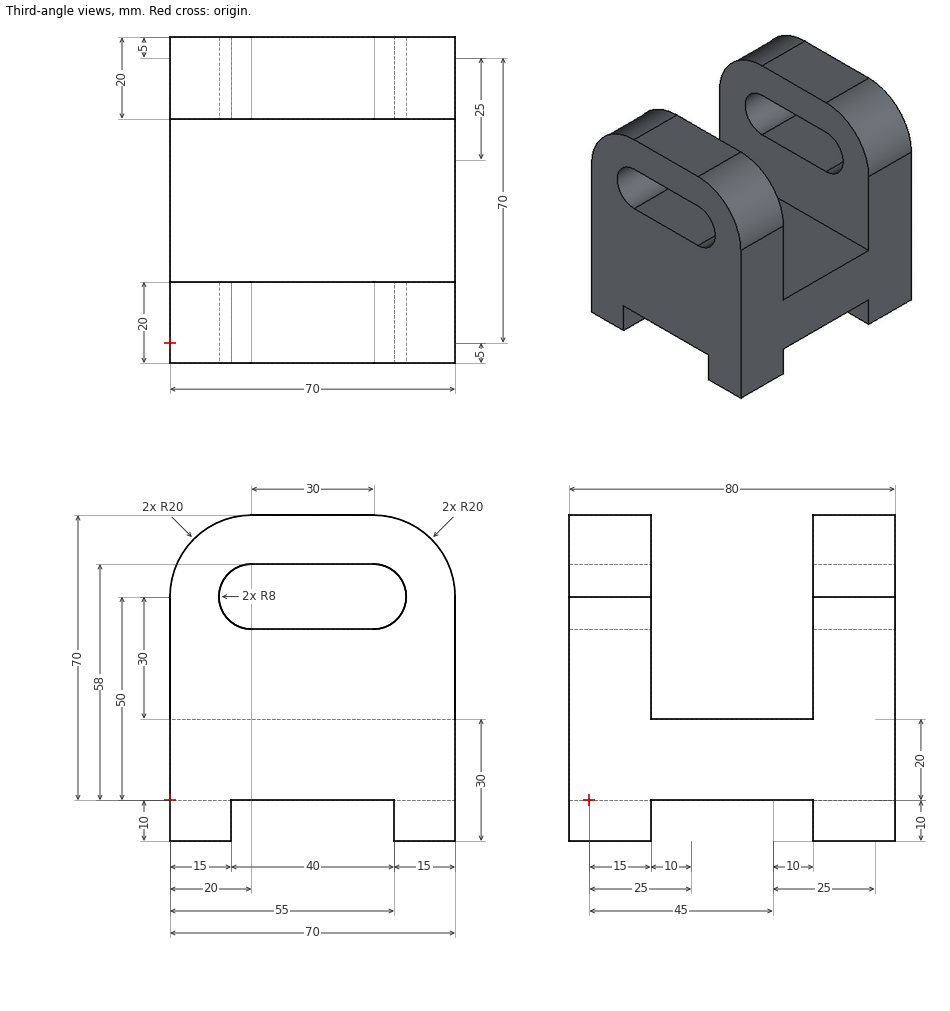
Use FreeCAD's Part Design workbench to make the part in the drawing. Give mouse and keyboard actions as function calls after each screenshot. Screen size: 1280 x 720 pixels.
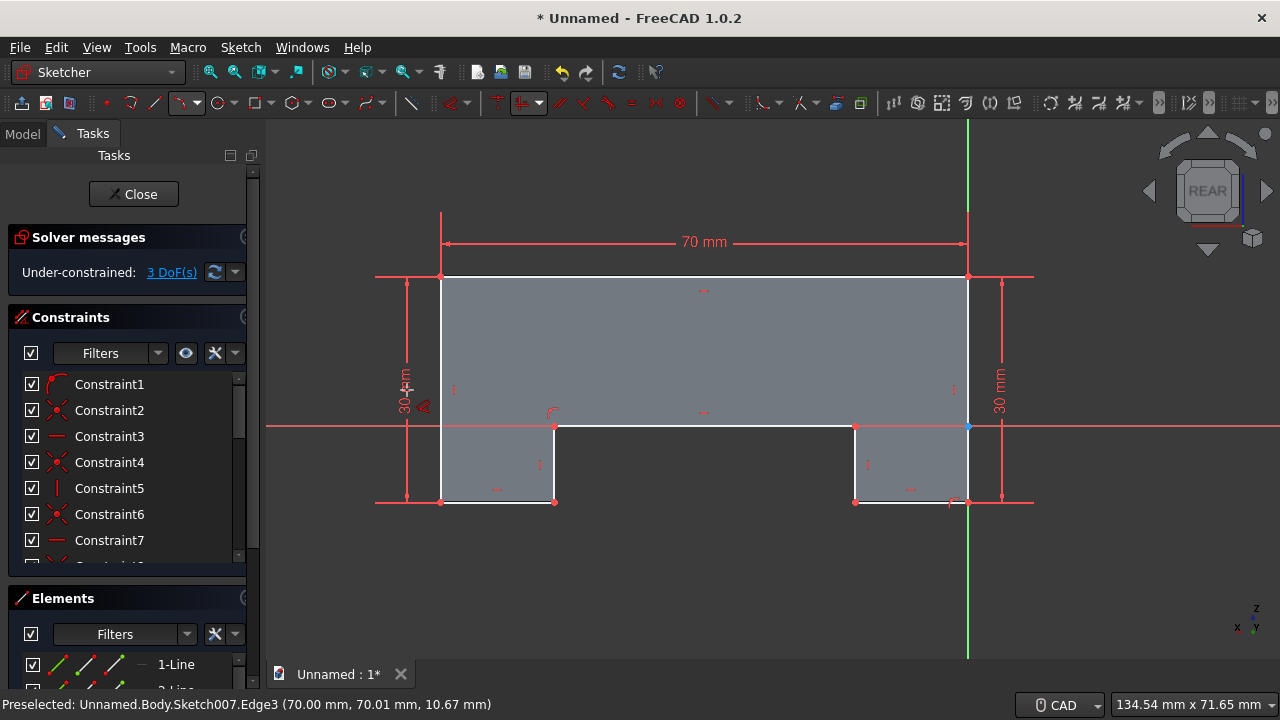
click(475, 503)
click(497, 537)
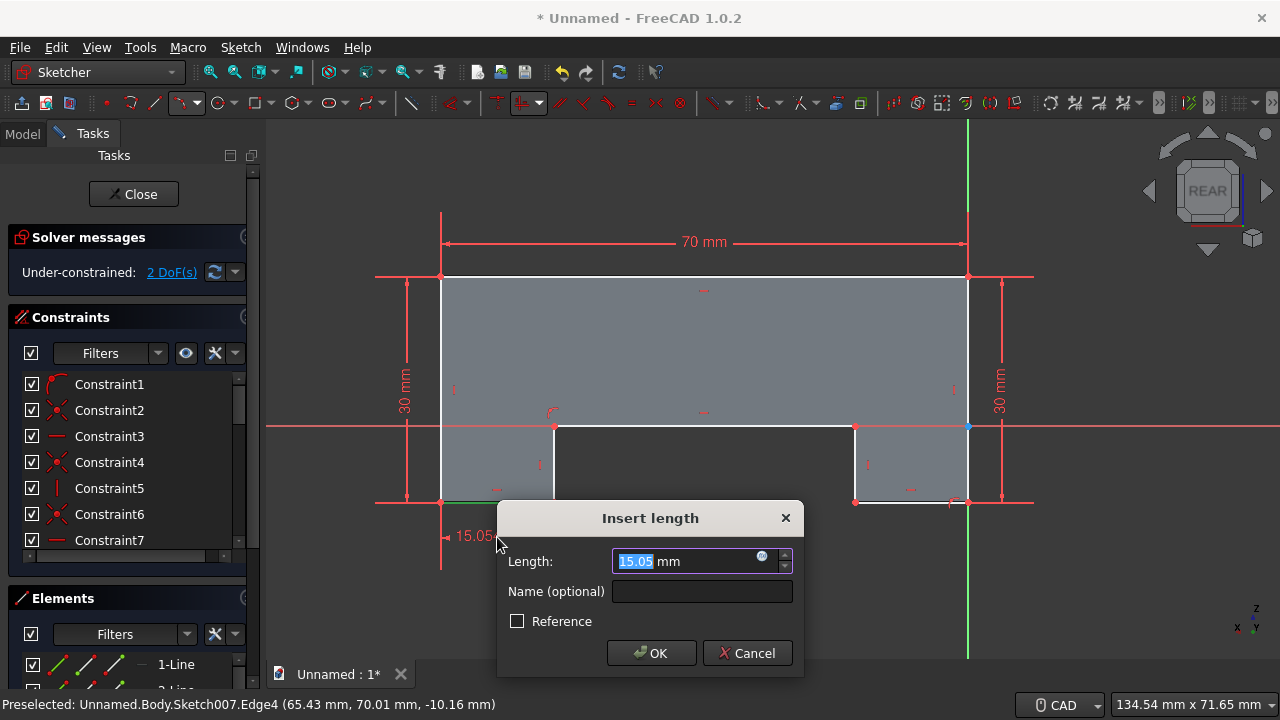
text(15)
key(Return)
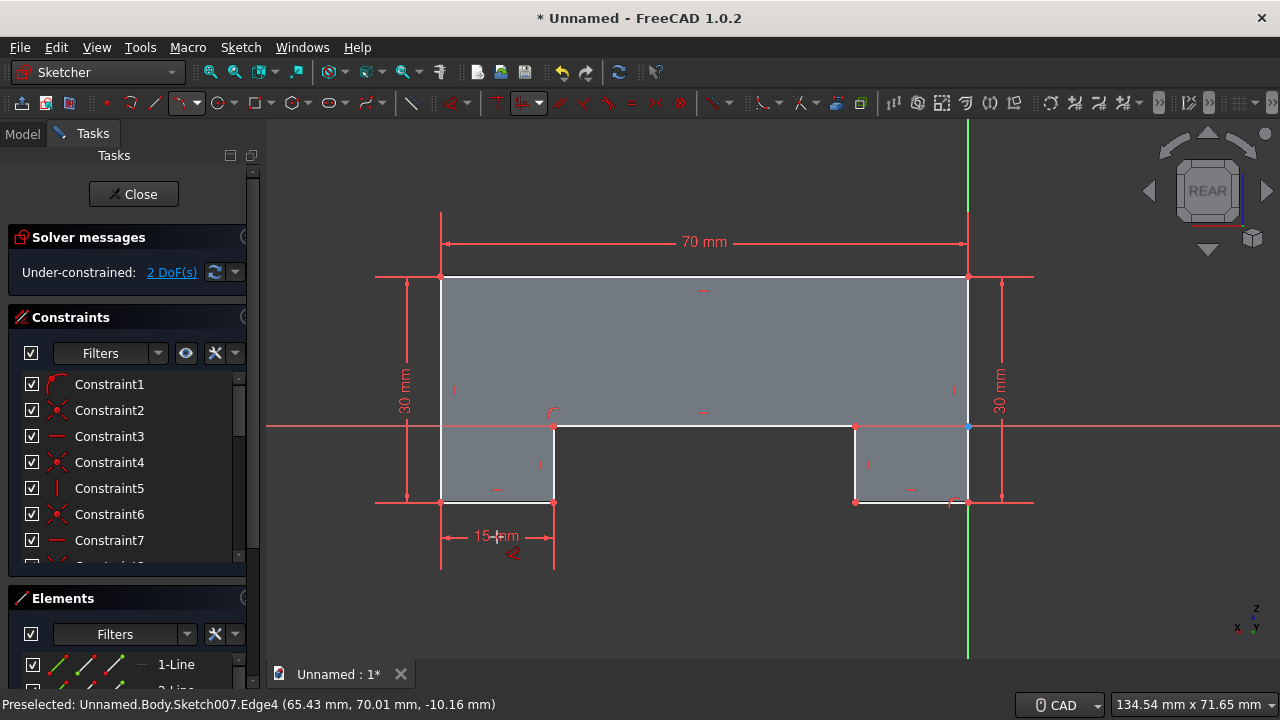
click(554, 480)
click(520, 465)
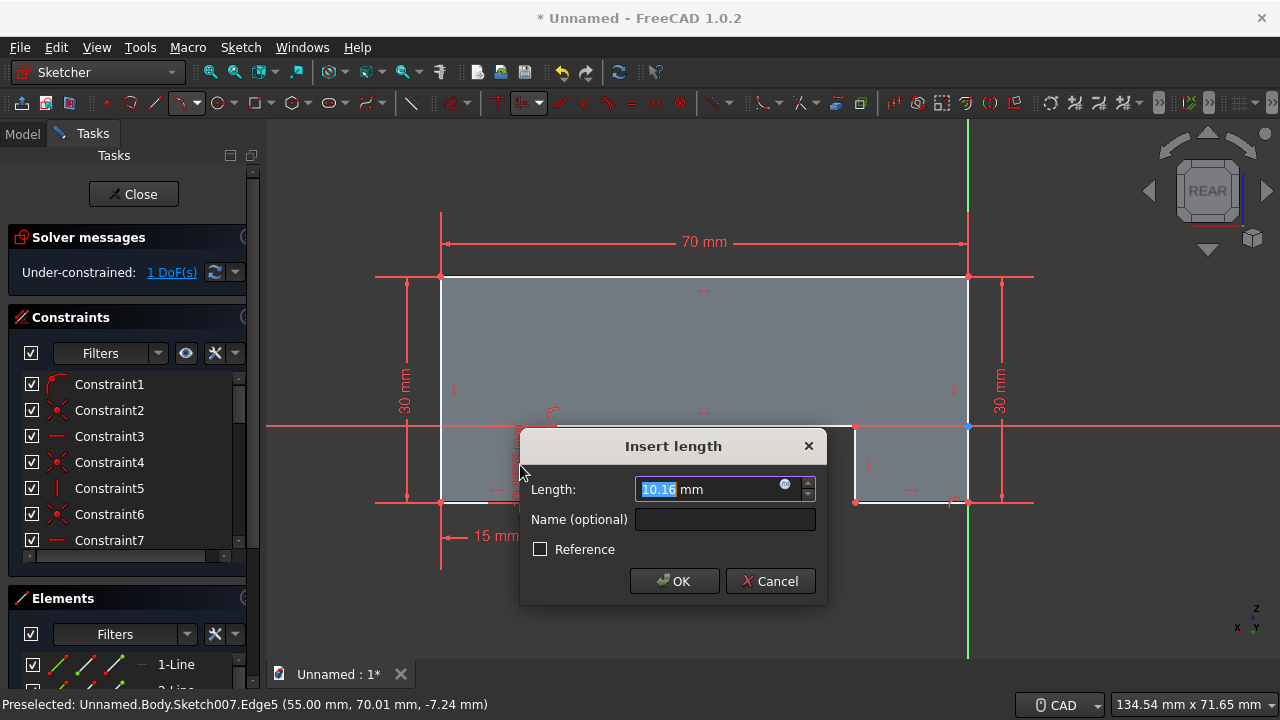
text(10)
key(Return)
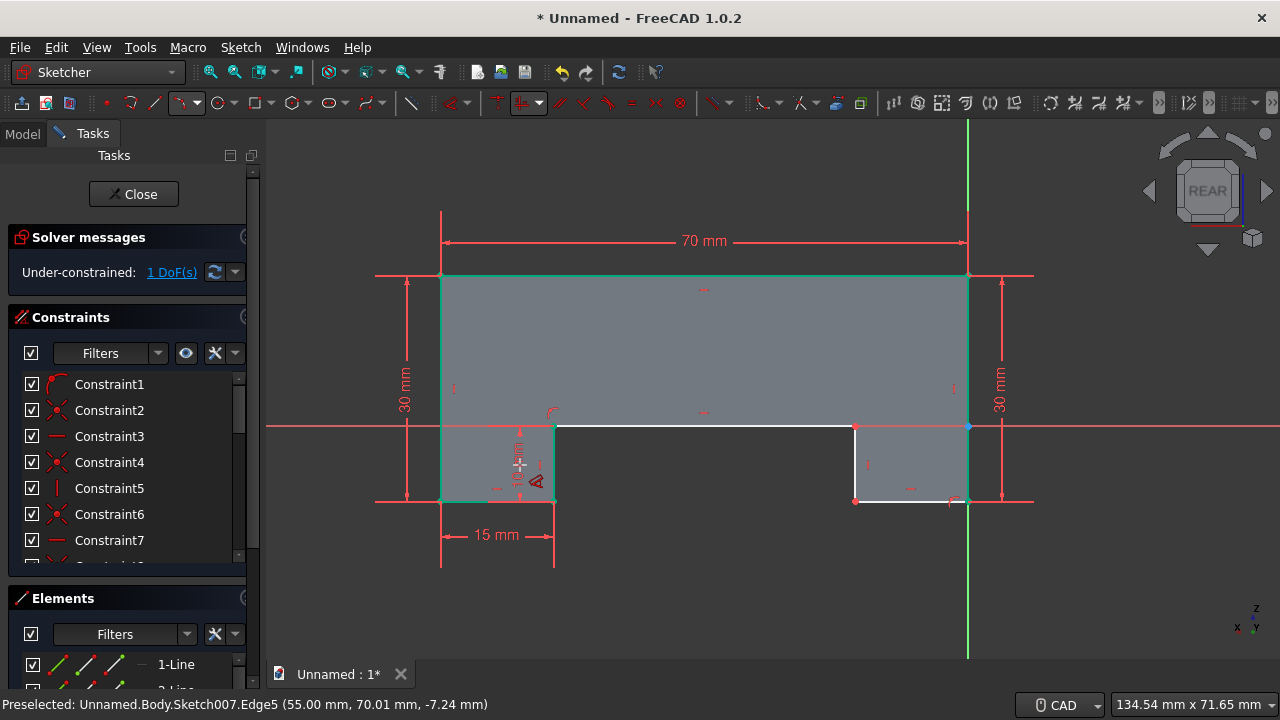
click(644, 426)
click(704, 460)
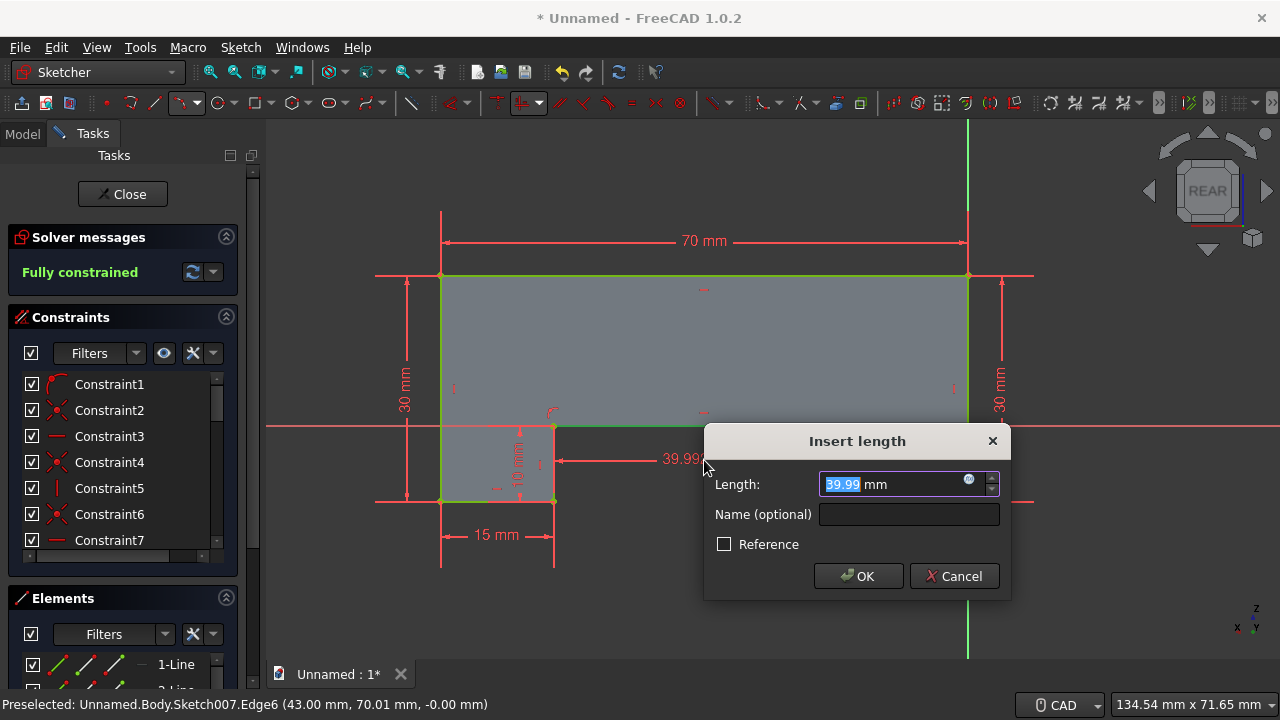
text(40)
key(Return)
key(Escape)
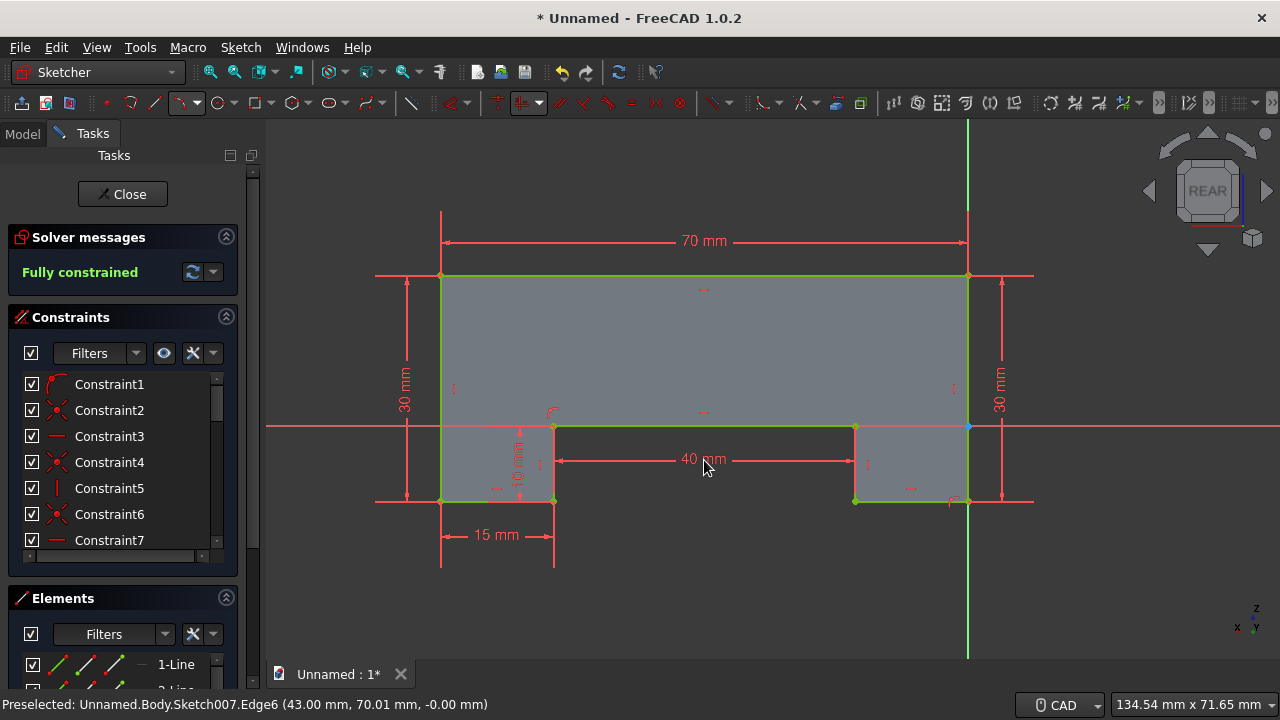
click(123, 194)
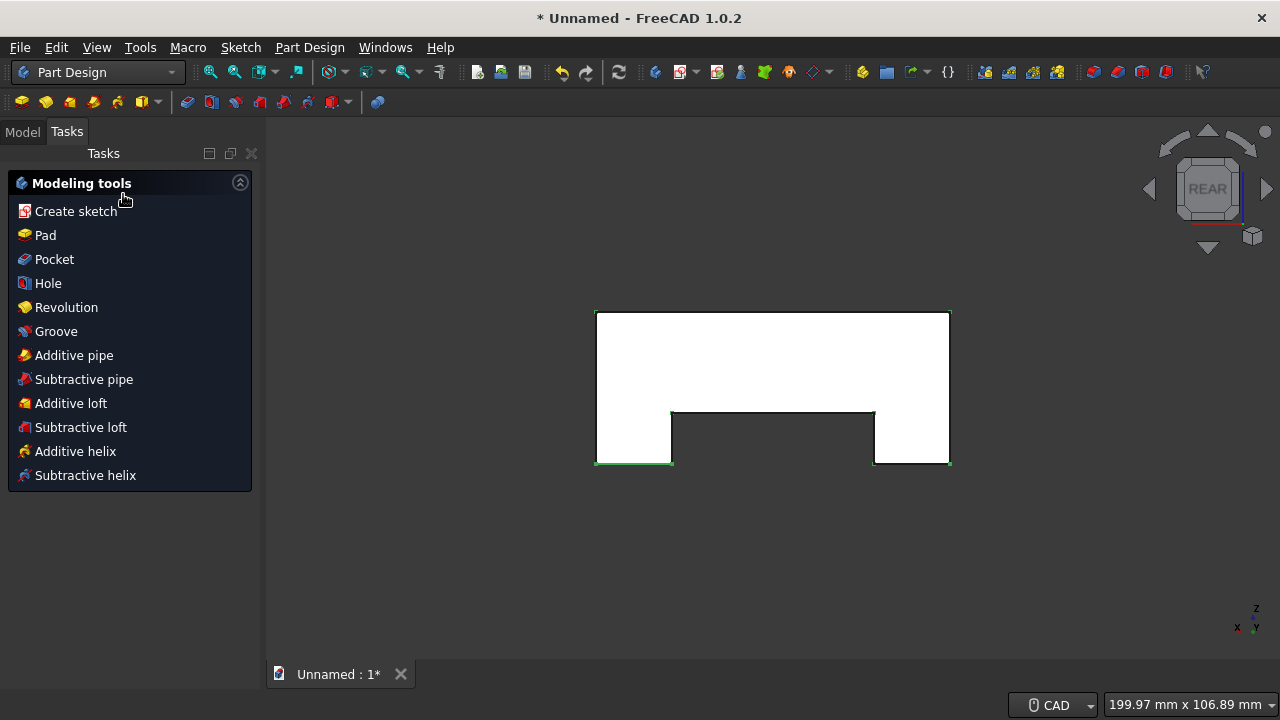
click(22, 102)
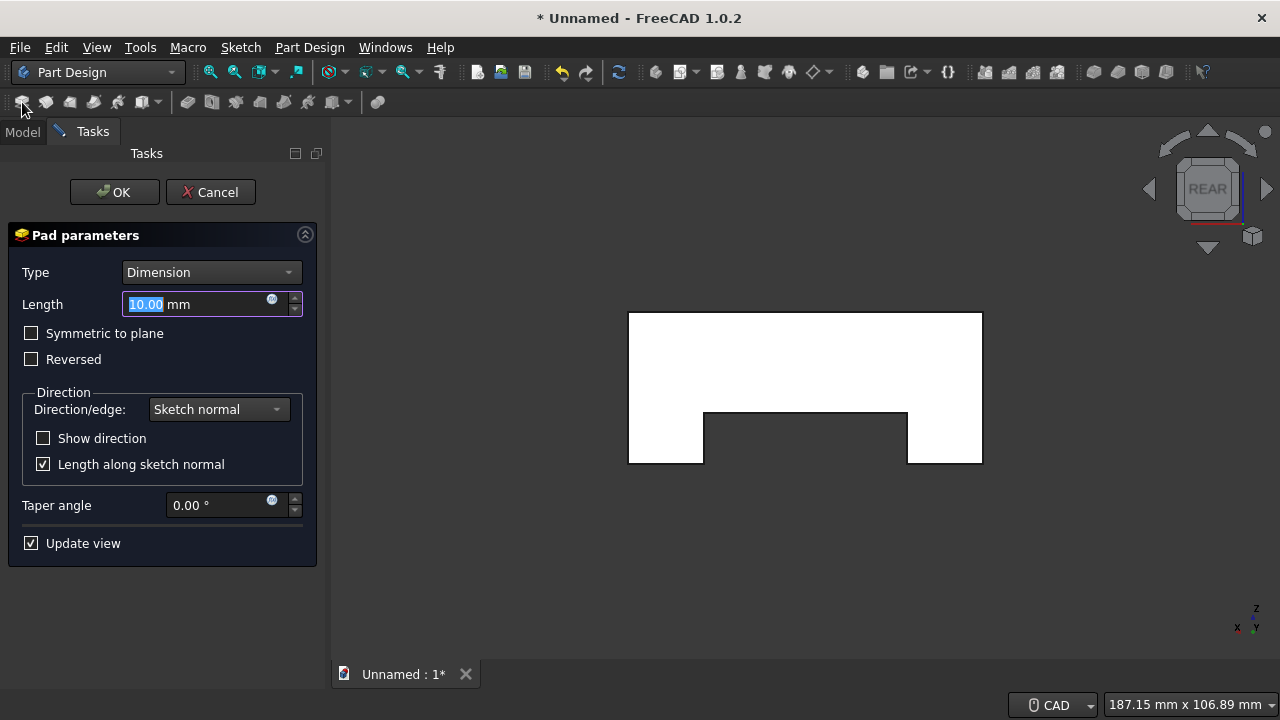
text(5)
key(Tab)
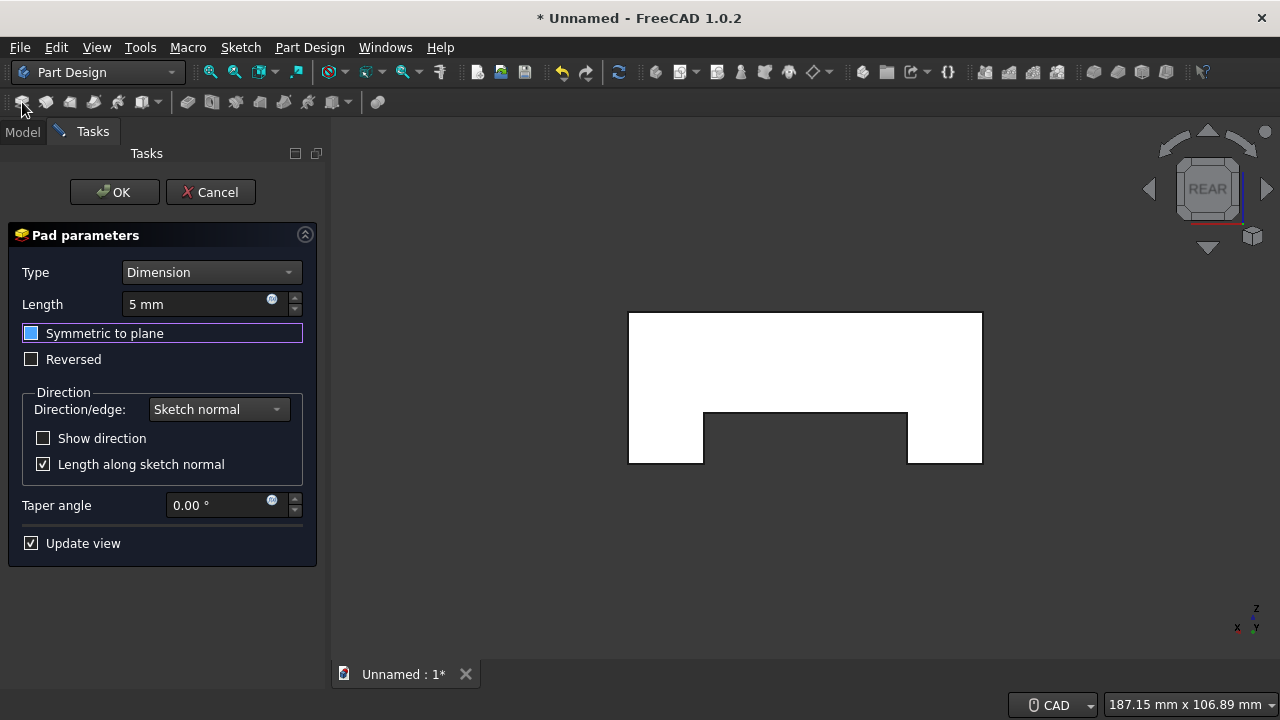
click(115, 192)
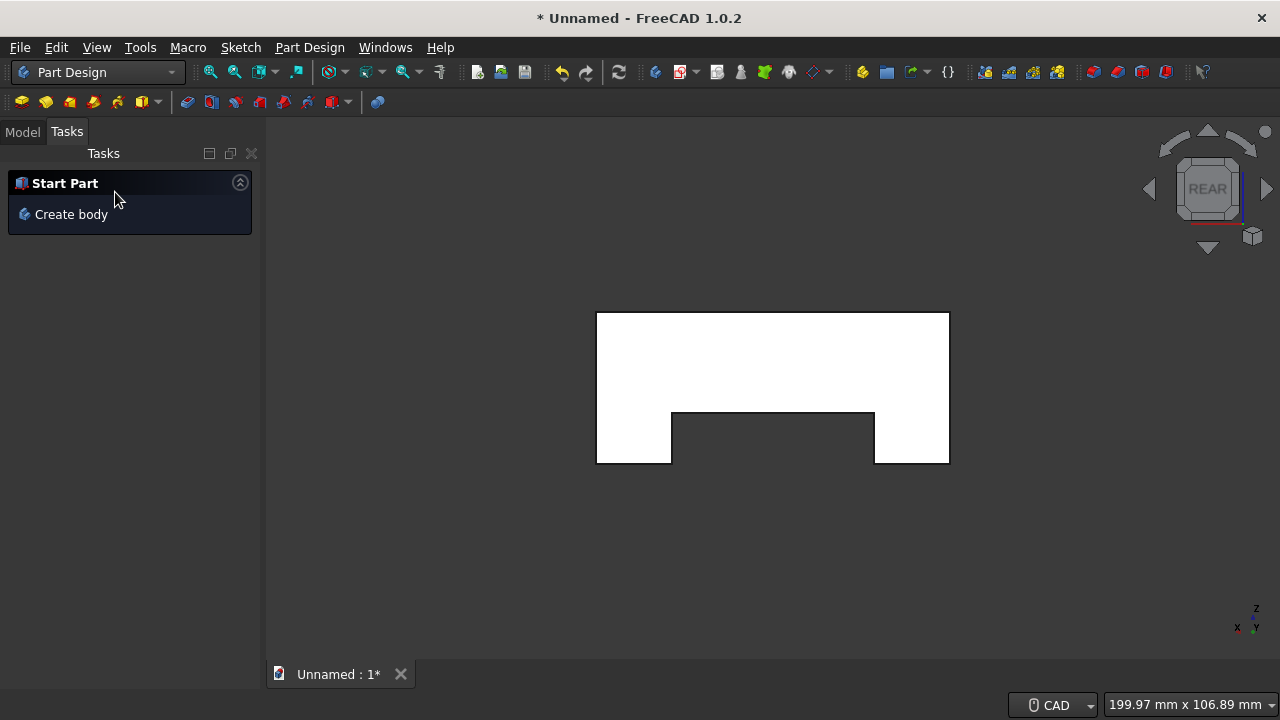
click(212, 72)